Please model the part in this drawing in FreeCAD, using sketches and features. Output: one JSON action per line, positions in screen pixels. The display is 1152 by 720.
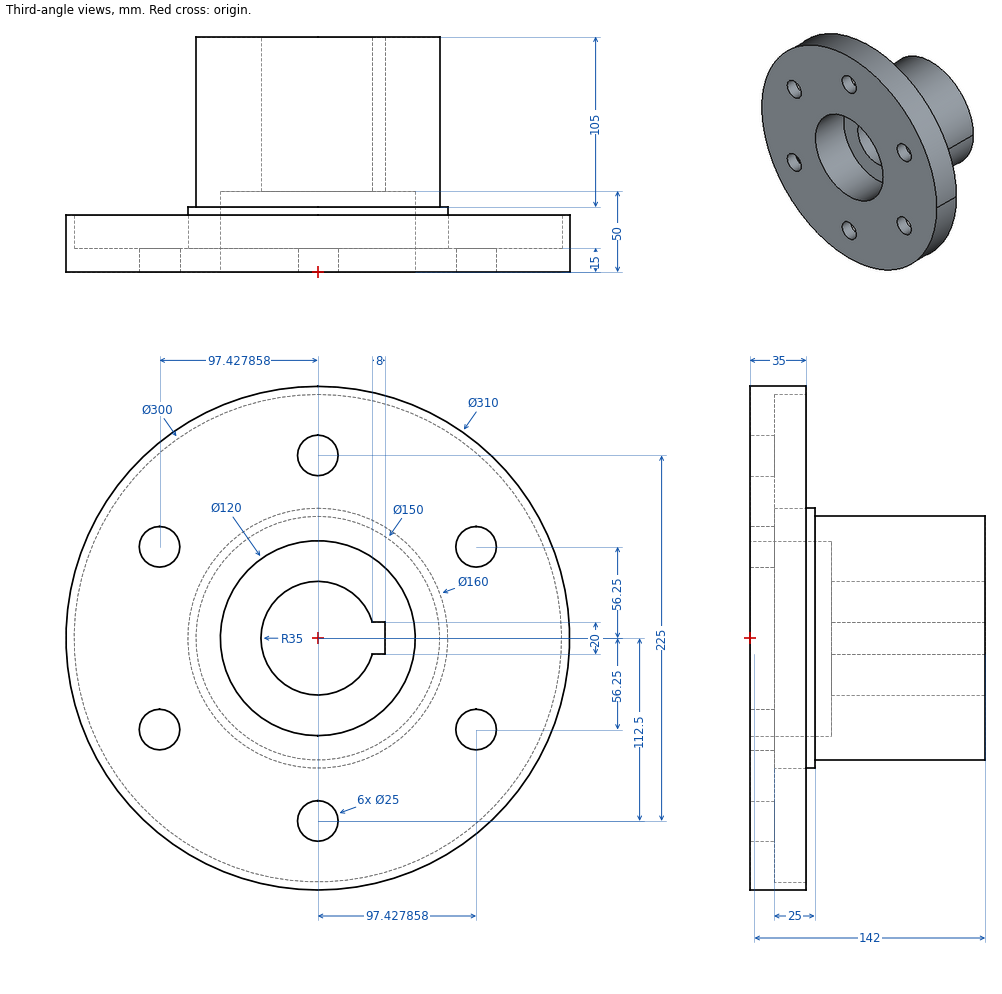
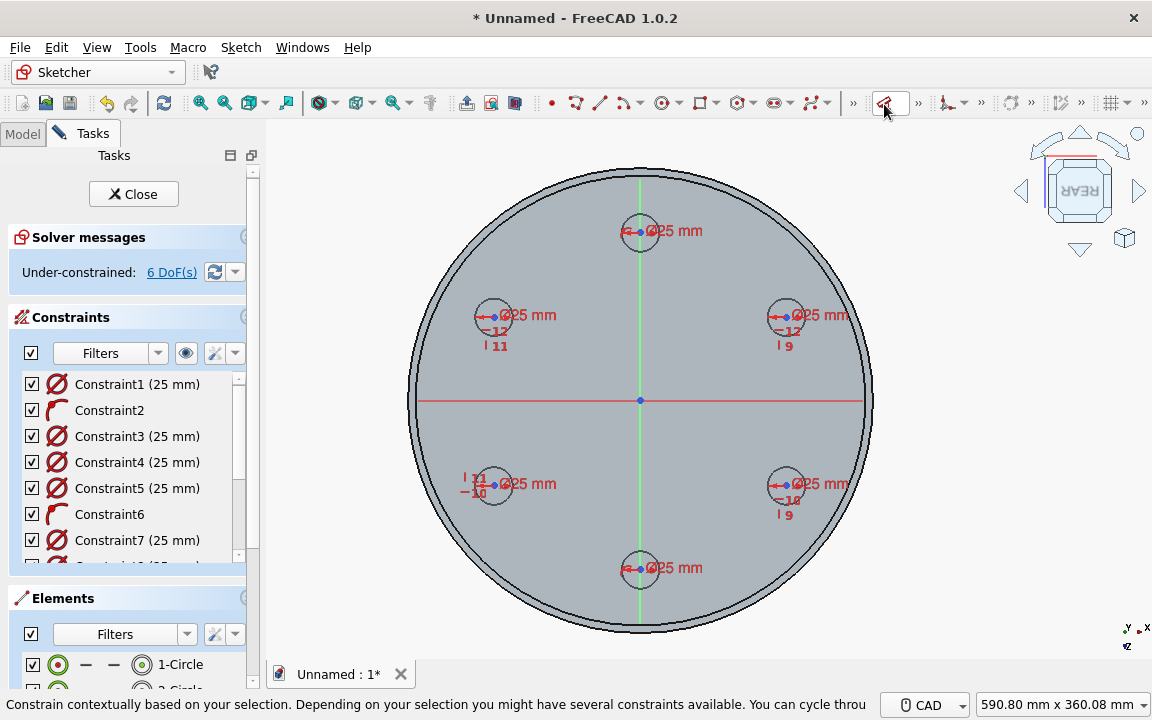
{"action": "left_click", "coordinate": [640, 233]}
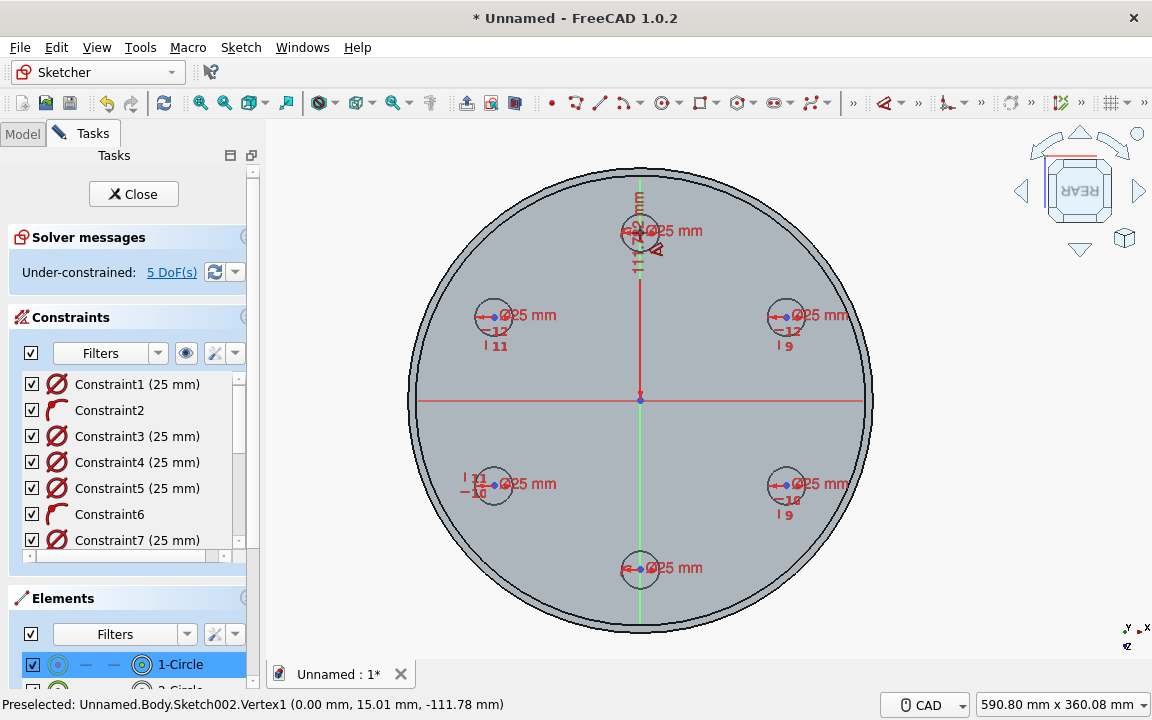
{"action": "left_click", "coordinate": [640, 570]}
{"action": "left_click", "coordinate": [674, 324]}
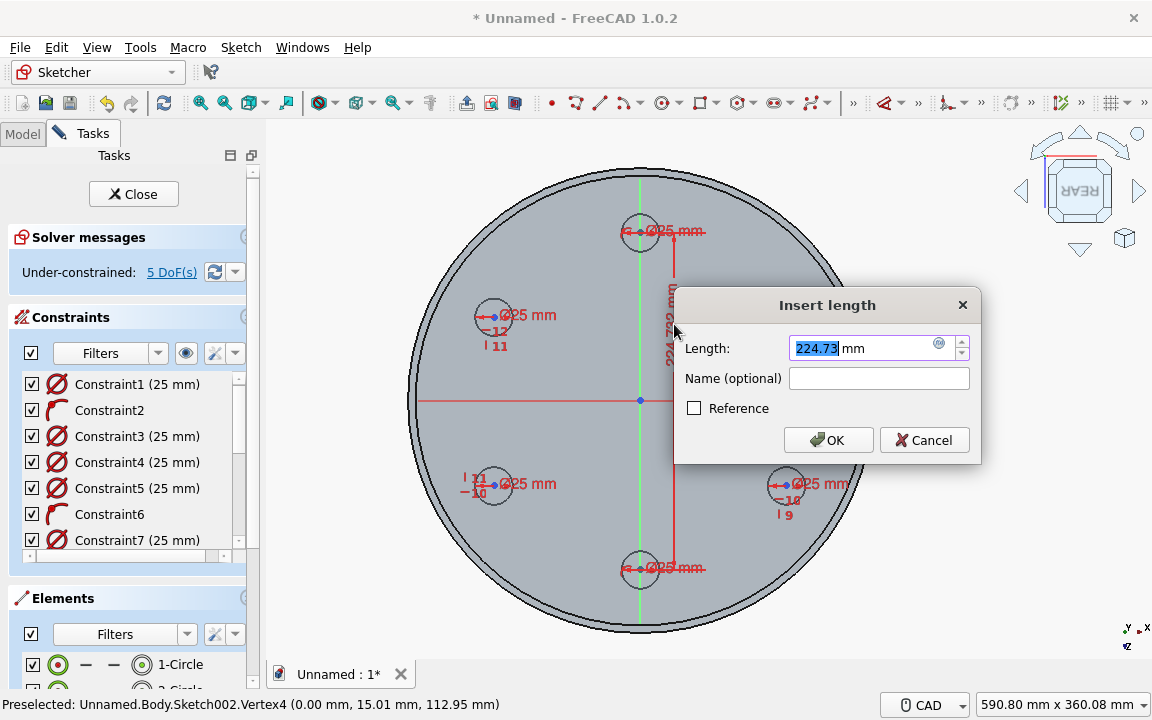
{"action": "type", "text": "225"}
{"action": "key", "text": "Return"}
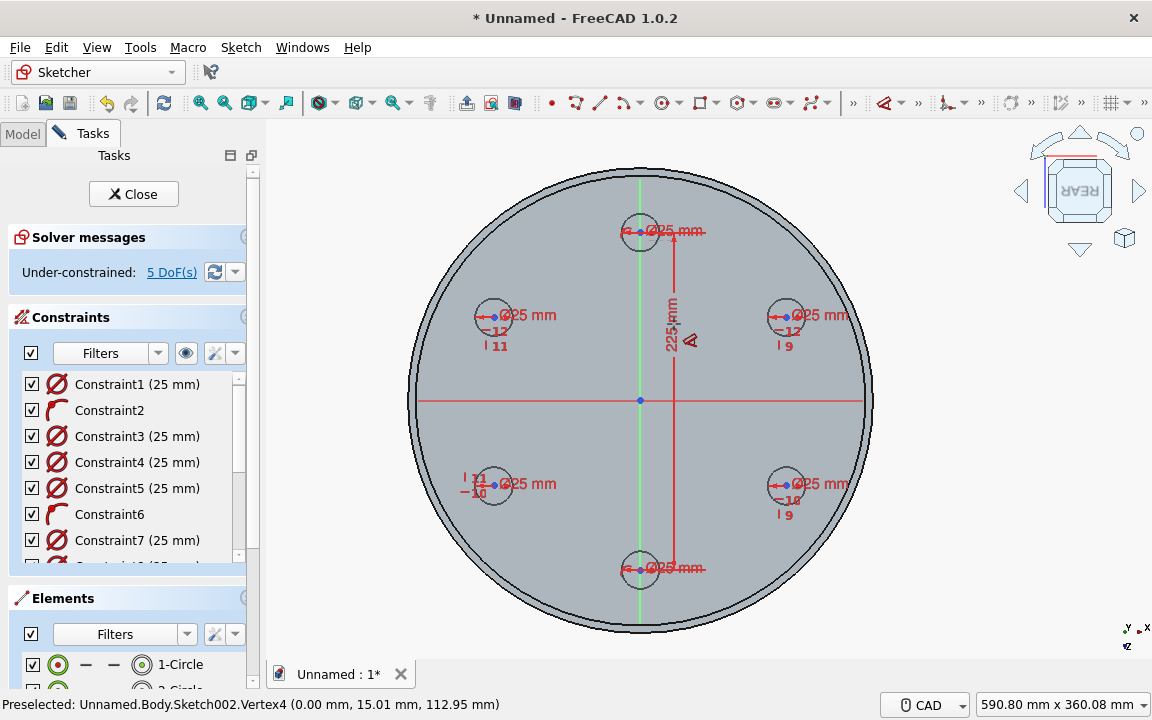
{"action": "left_click", "coordinate": [640, 233]}
{"action": "left_click", "coordinate": [674, 278]}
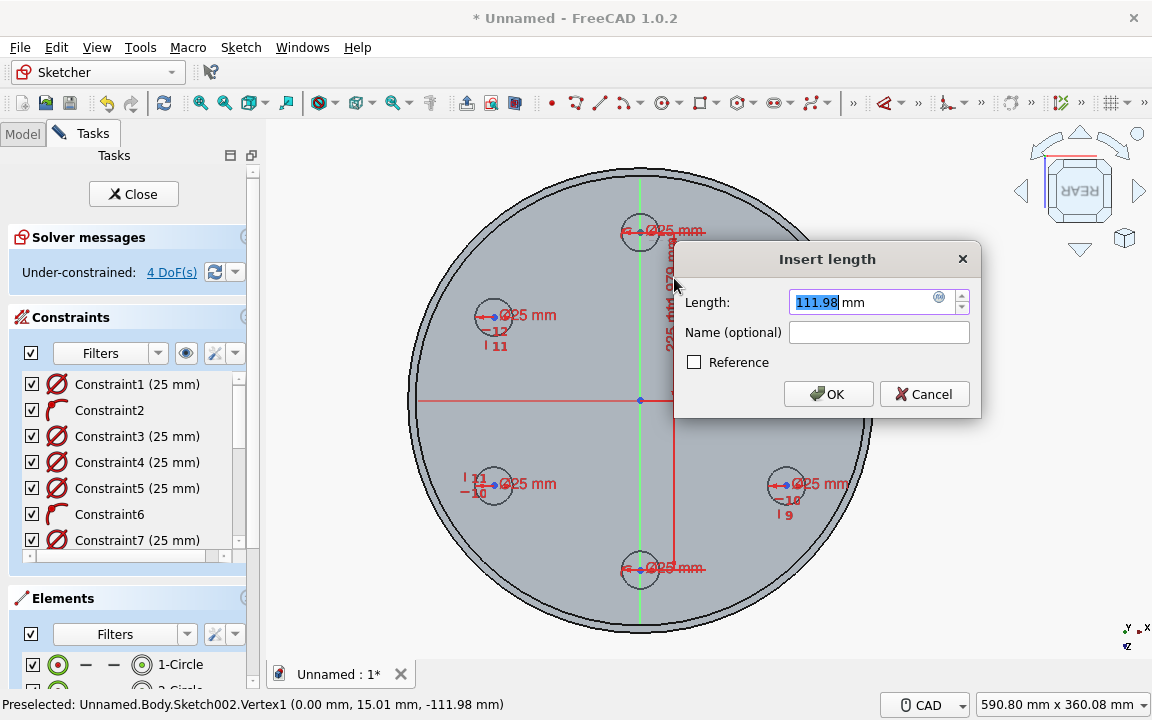
{"action": "type", "text": "112.5"}
{"action": "key", "text": "Return"}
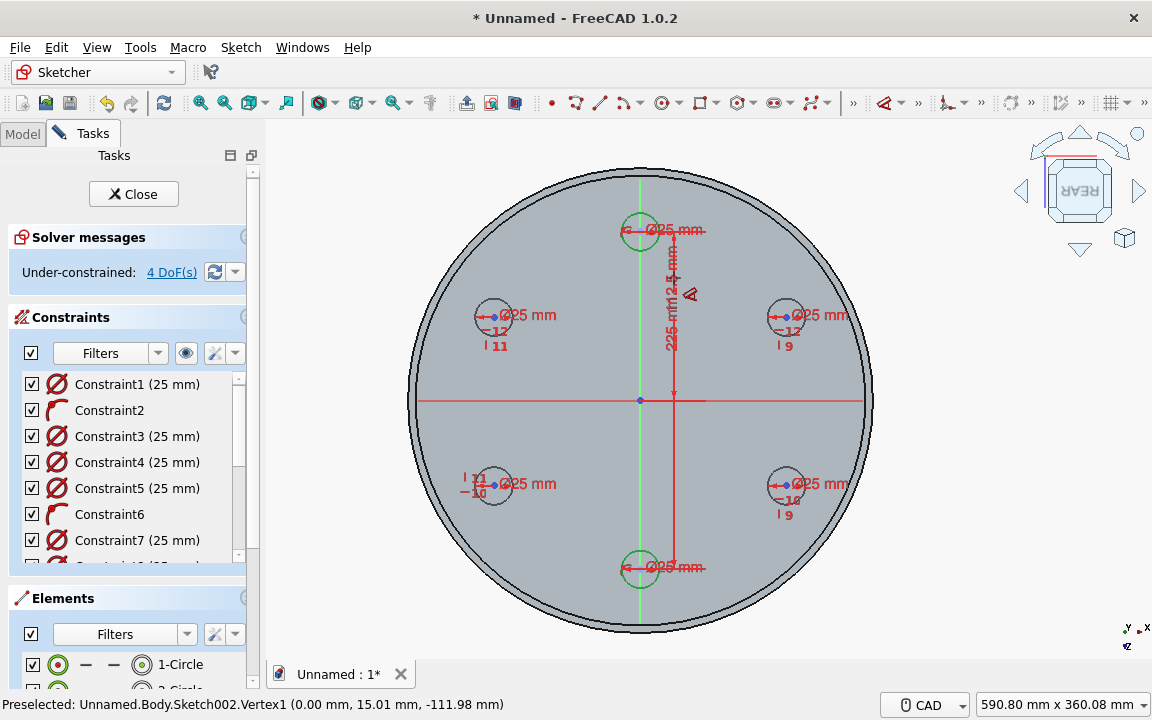
{"action": "left_click", "coordinate": [786, 317]}
{"action": "left_click", "coordinate": [820, 359]}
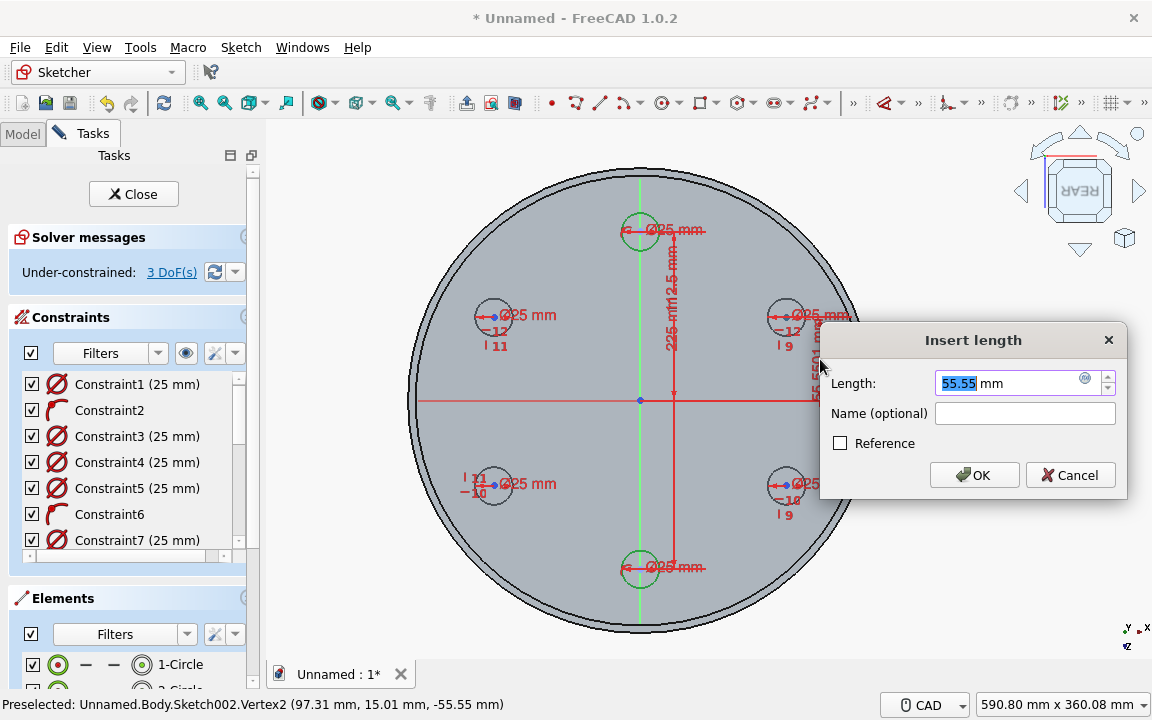
{"action": "type", "text": "56.25"}
{"action": "key", "text": "Return"}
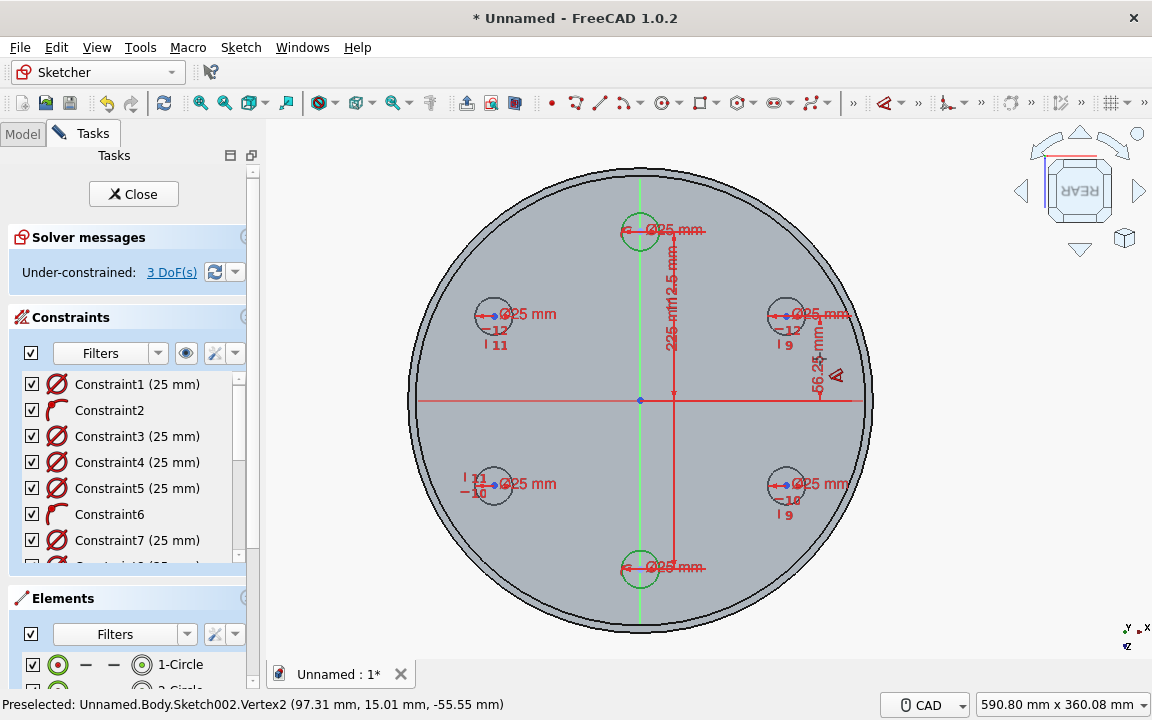
{"action": "left_click", "coordinate": [786, 486]}
{"action": "left_click", "coordinate": [820, 443]}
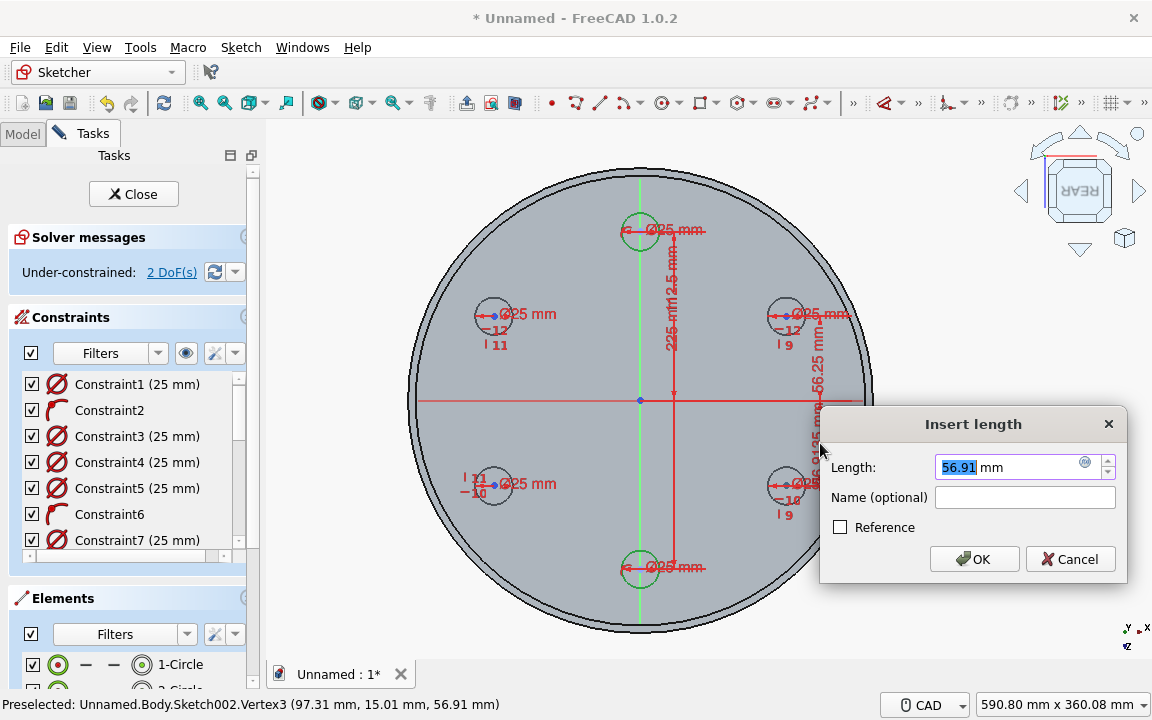
{"action": "type", "text": "56.25"}
{"action": "key", "text": "Return"}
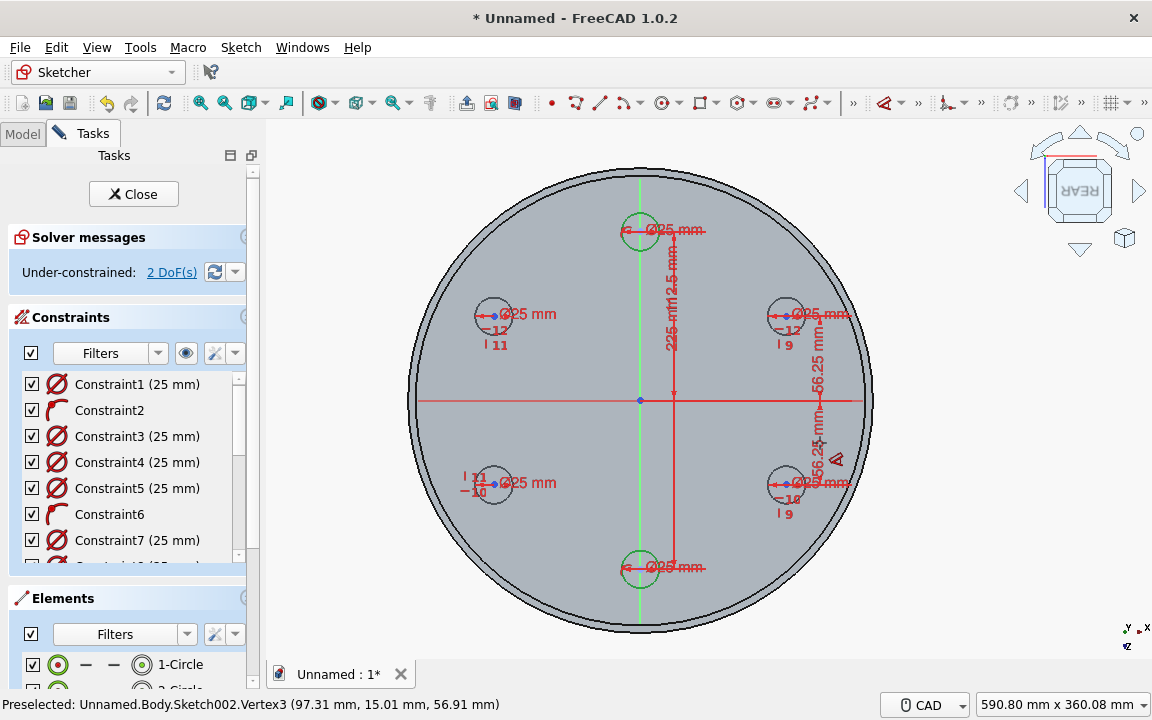
{"action": "left_click", "coordinate": [786, 316]}
{"action": "left_click", "coordinate": [747, 282]}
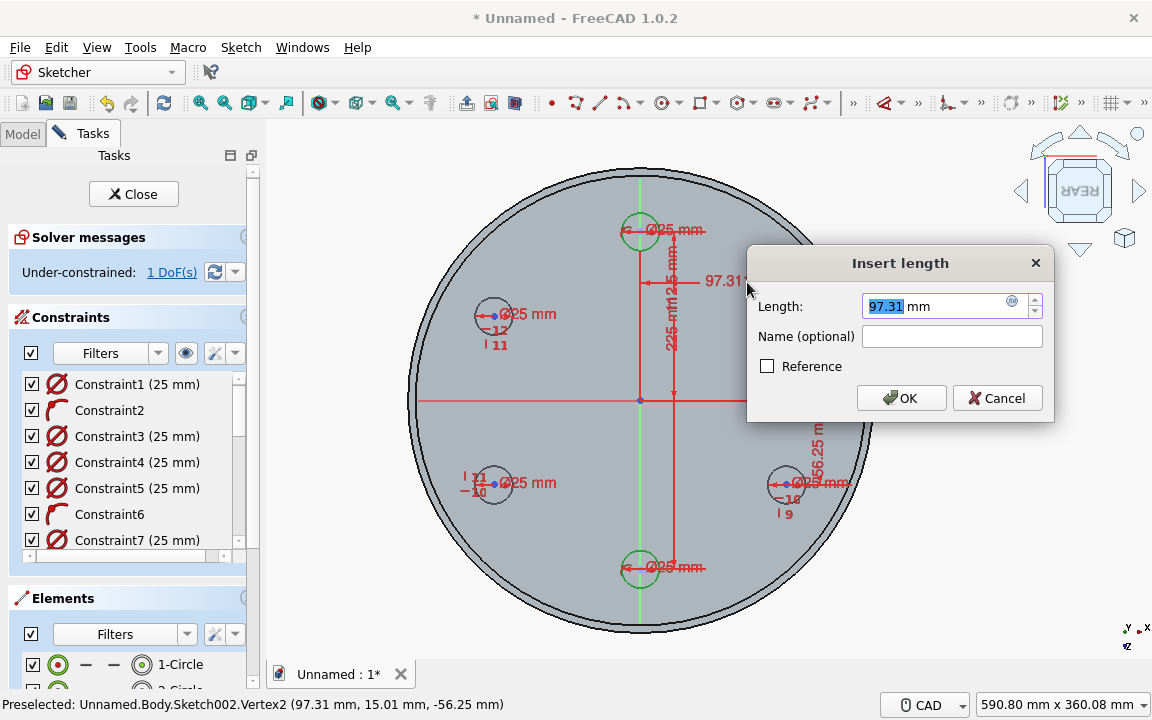
{"action": "type", "text": "97.427858"}
{"action": "key", "text": "Return"}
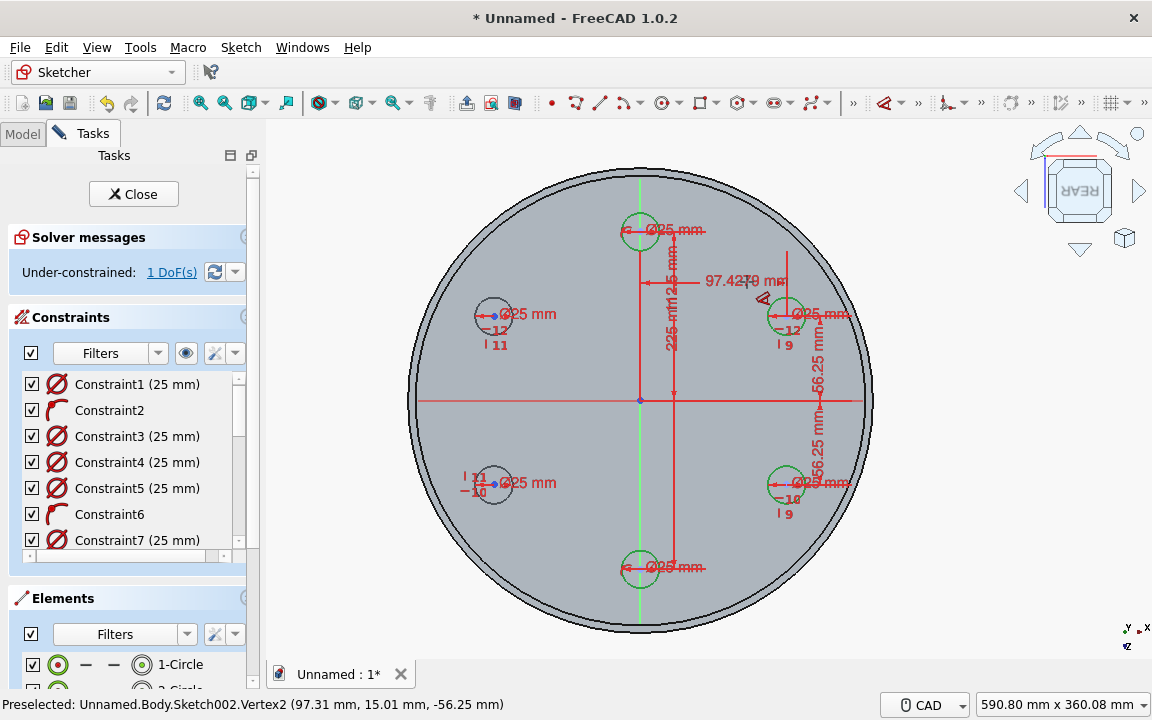
{"action": "left_click", "coordinate": [494, 485]}
{"action": "left_click", "coordinate": [567, 519]}